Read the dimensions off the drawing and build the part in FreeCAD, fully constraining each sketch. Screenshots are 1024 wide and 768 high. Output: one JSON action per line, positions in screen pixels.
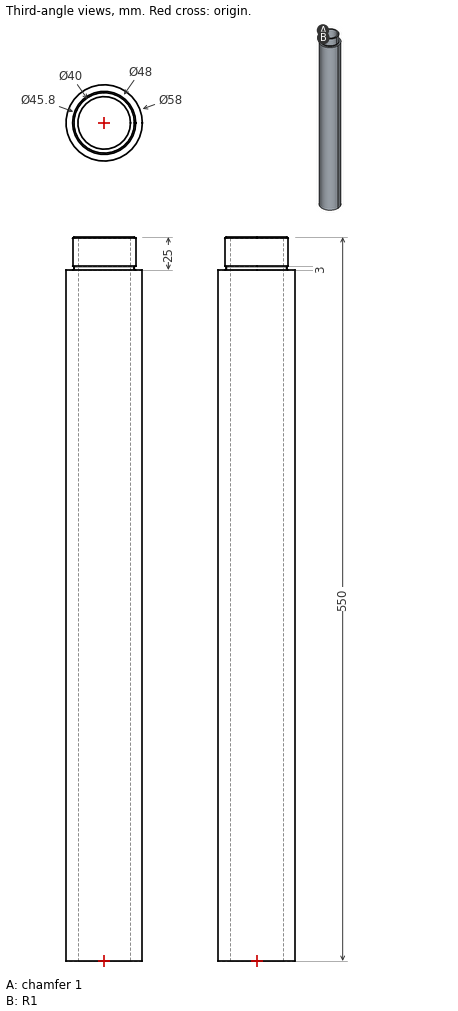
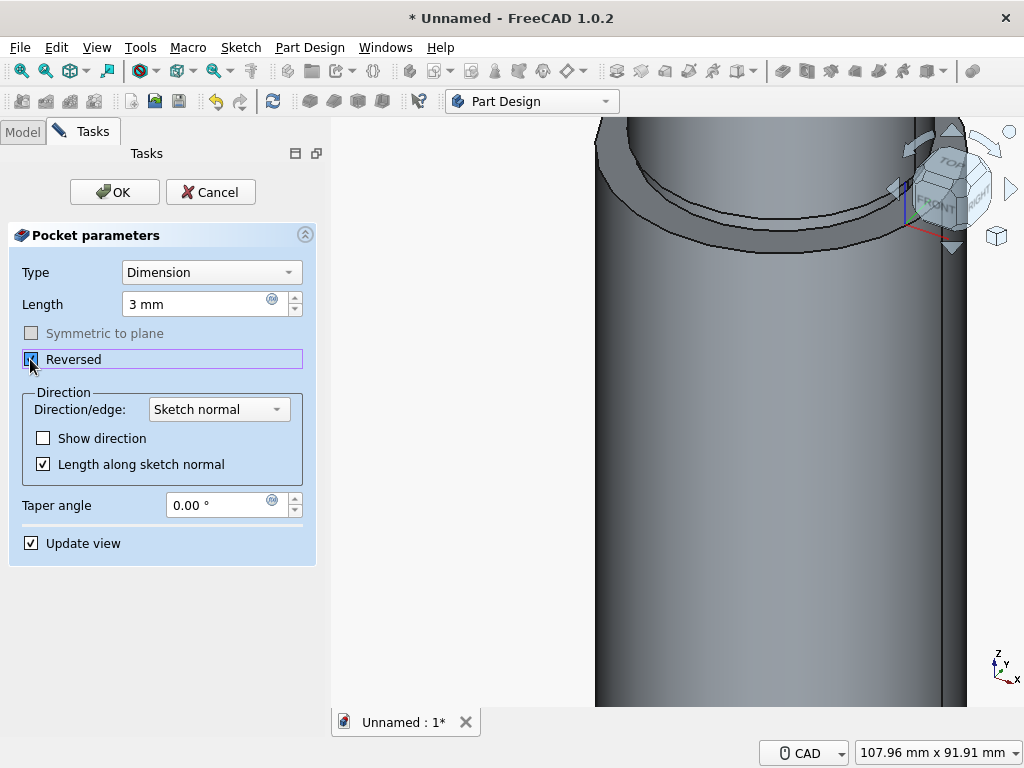
{"action": "left_click", "coordinate": [115, 192]}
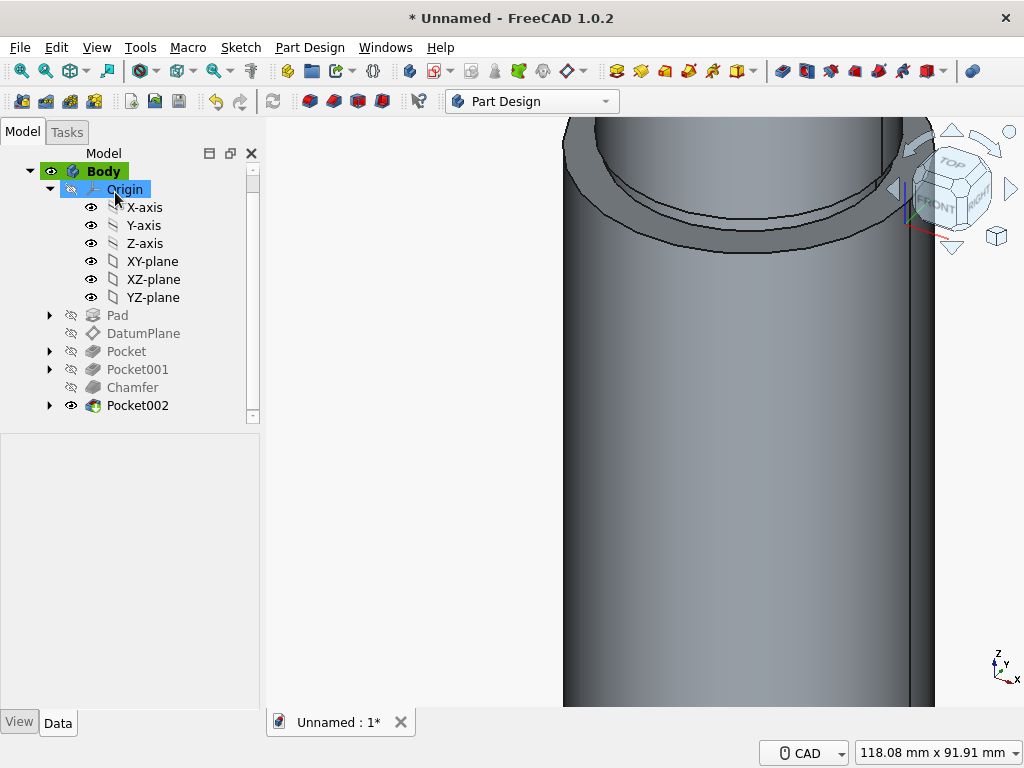
{"action": "left_click", "coordinate": [22, 72]}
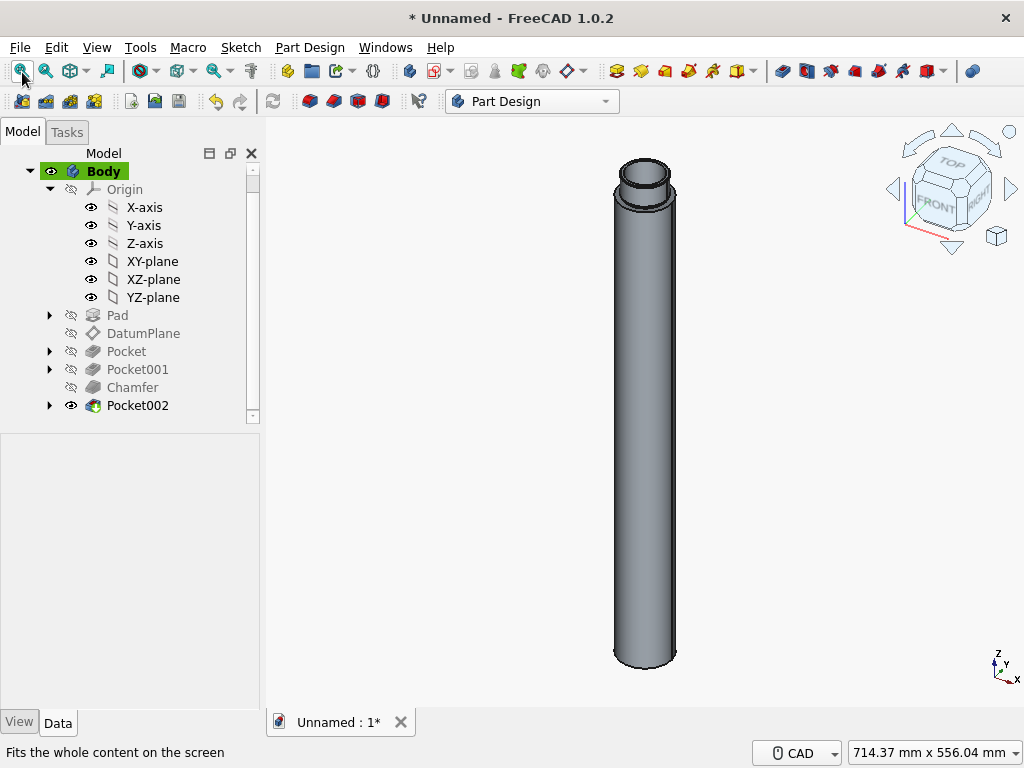
{"action": "key", "text": "0"}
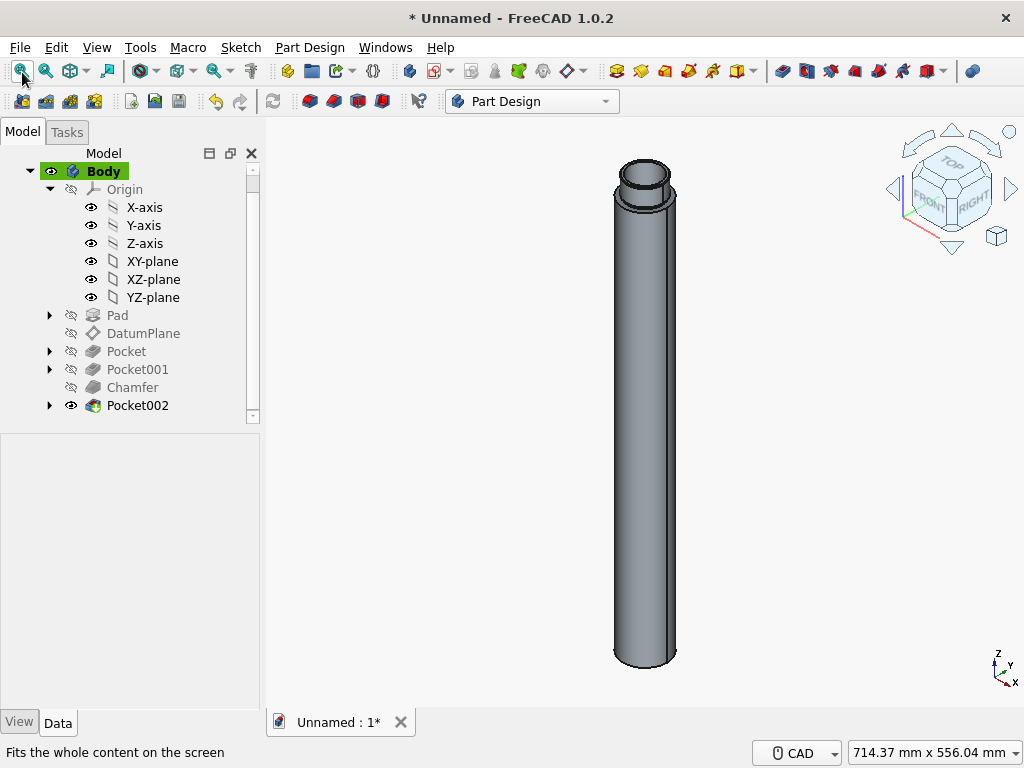
{"action": "key", "text": "2"}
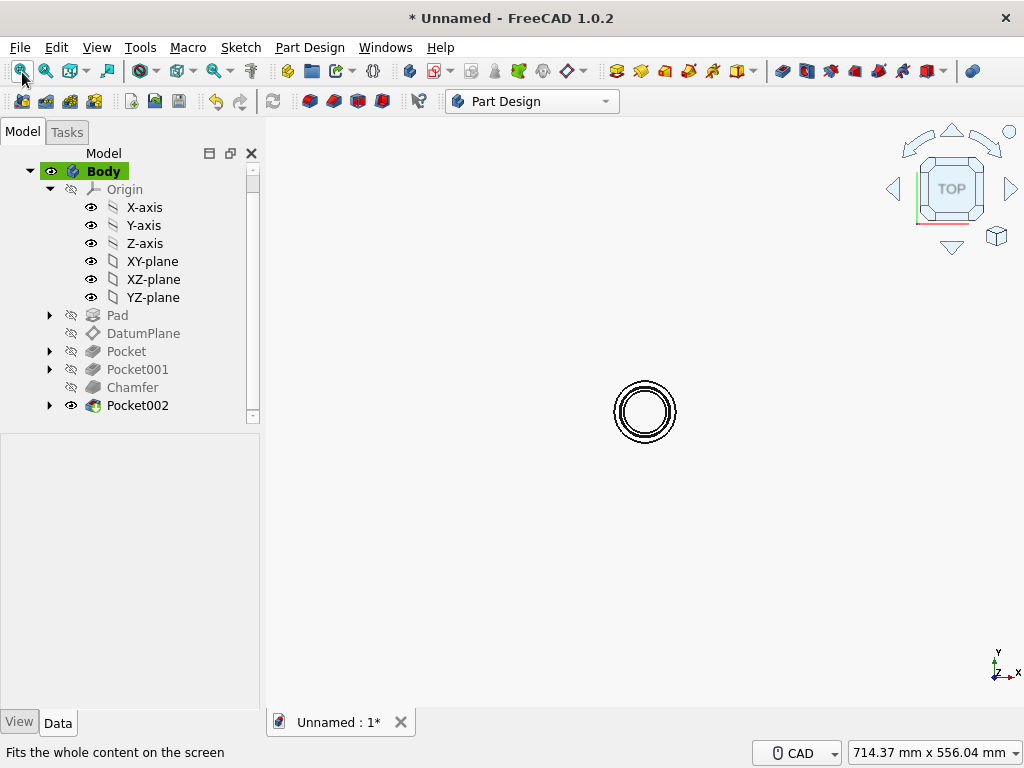
{"action": "left_click", "coordinate": [22, 72]}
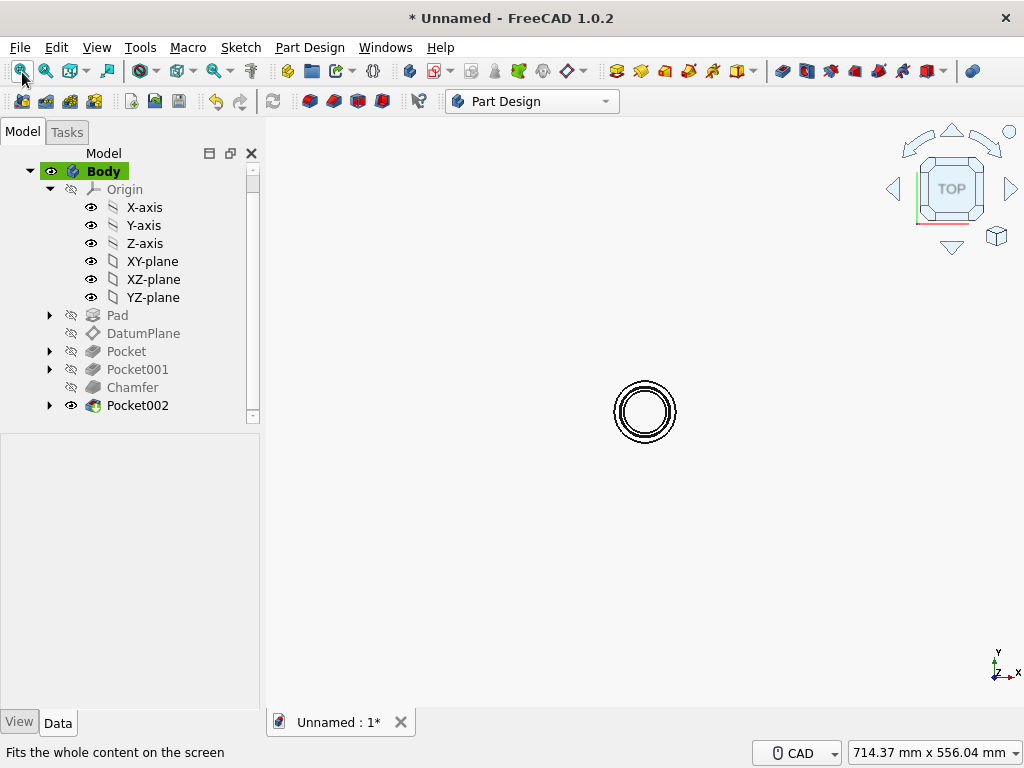
{"action": "key", "text": "1"}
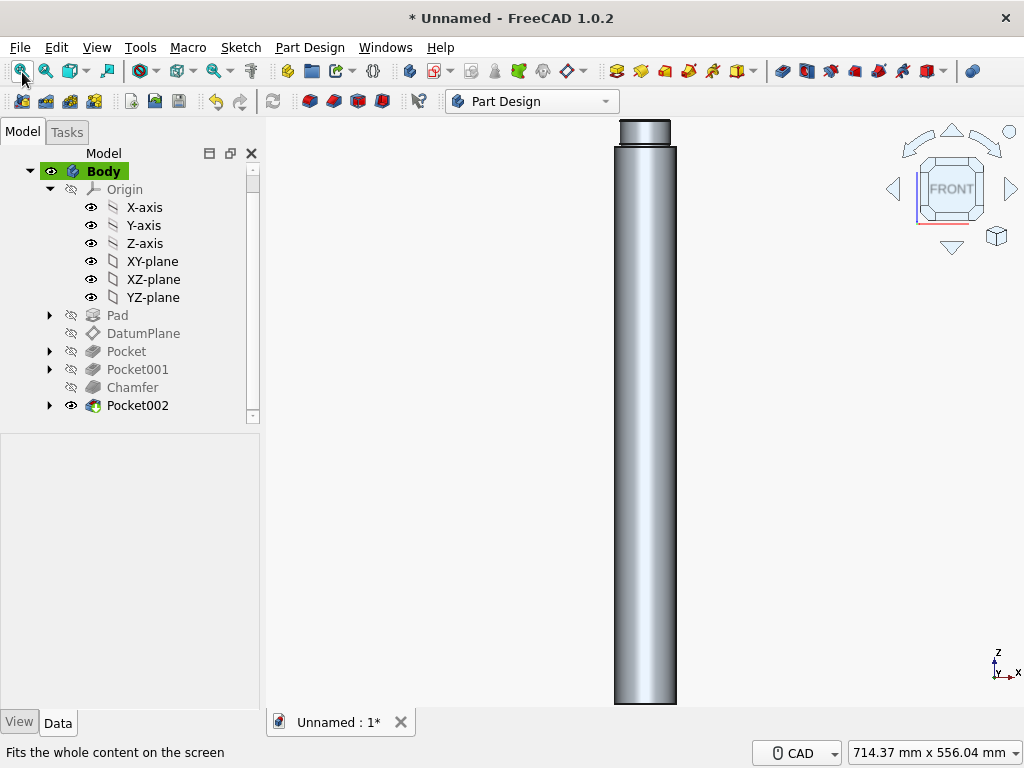
{"action": "key", "text": "3"}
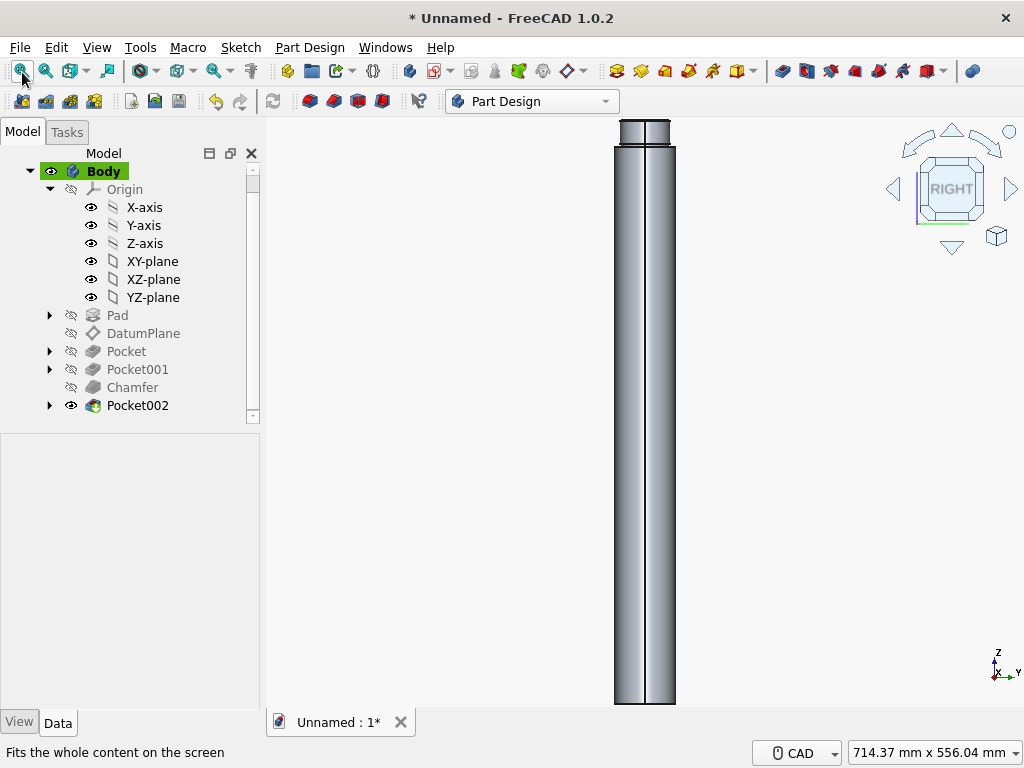
{"action": "key", "text": "5"}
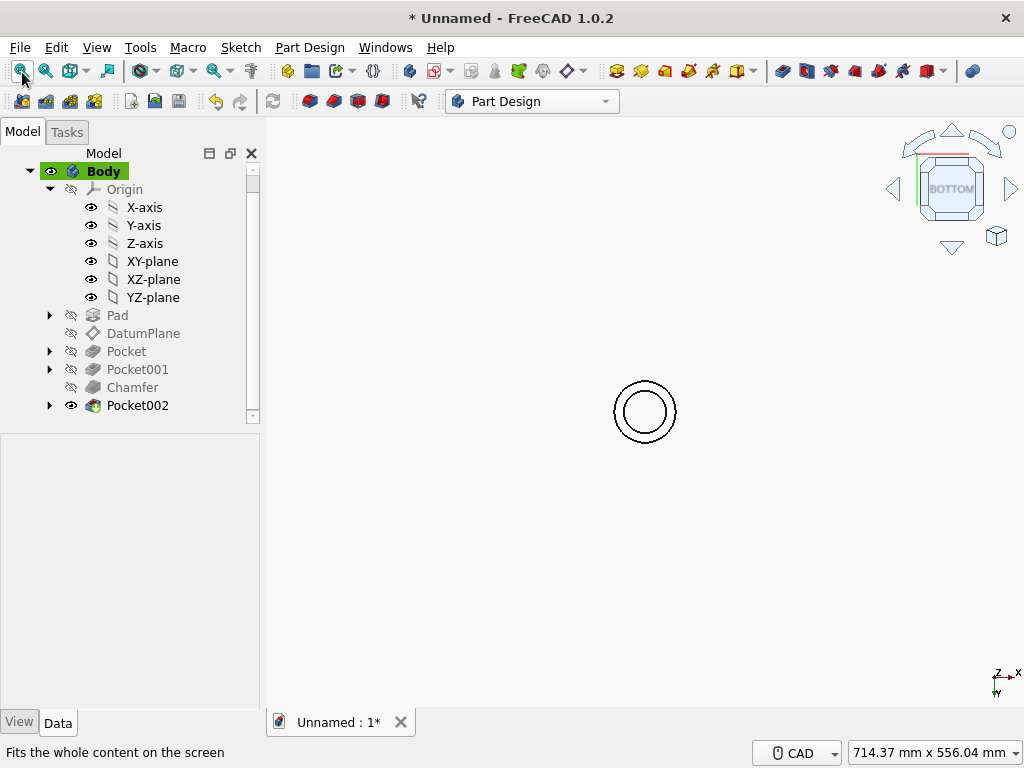
{"action": "left_click", "coordinate": [22, 72]}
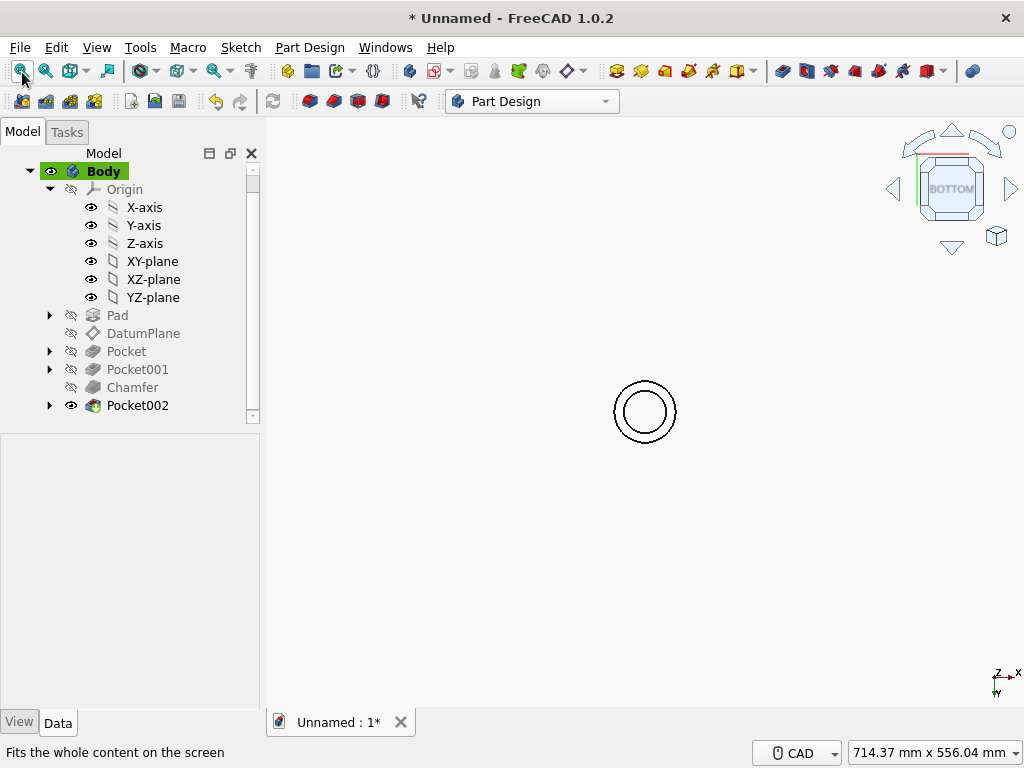
{"action": "key", "text": "4"}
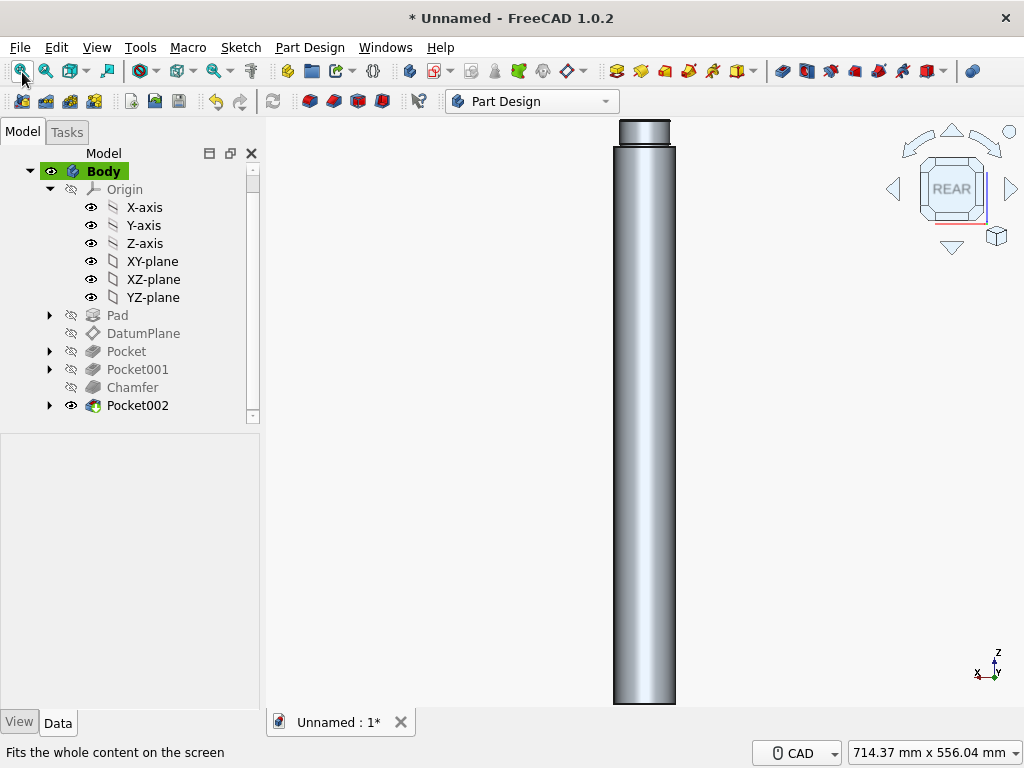
{"action": "key", "text": "6"}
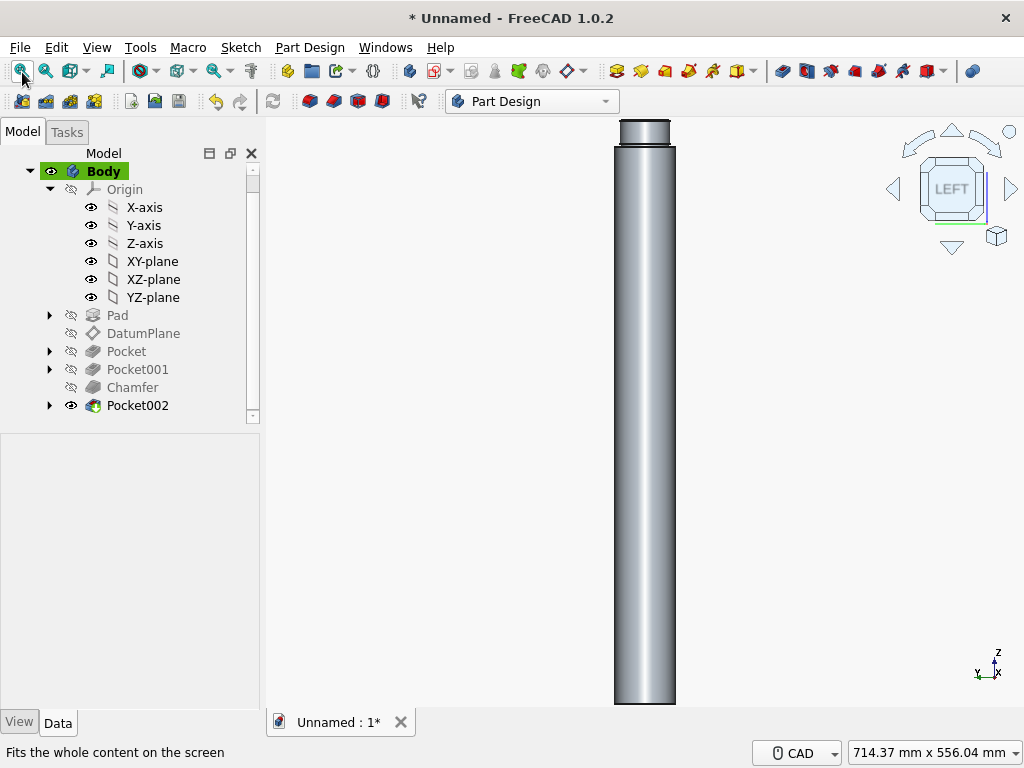
{"action": "key", "text": "v 3"}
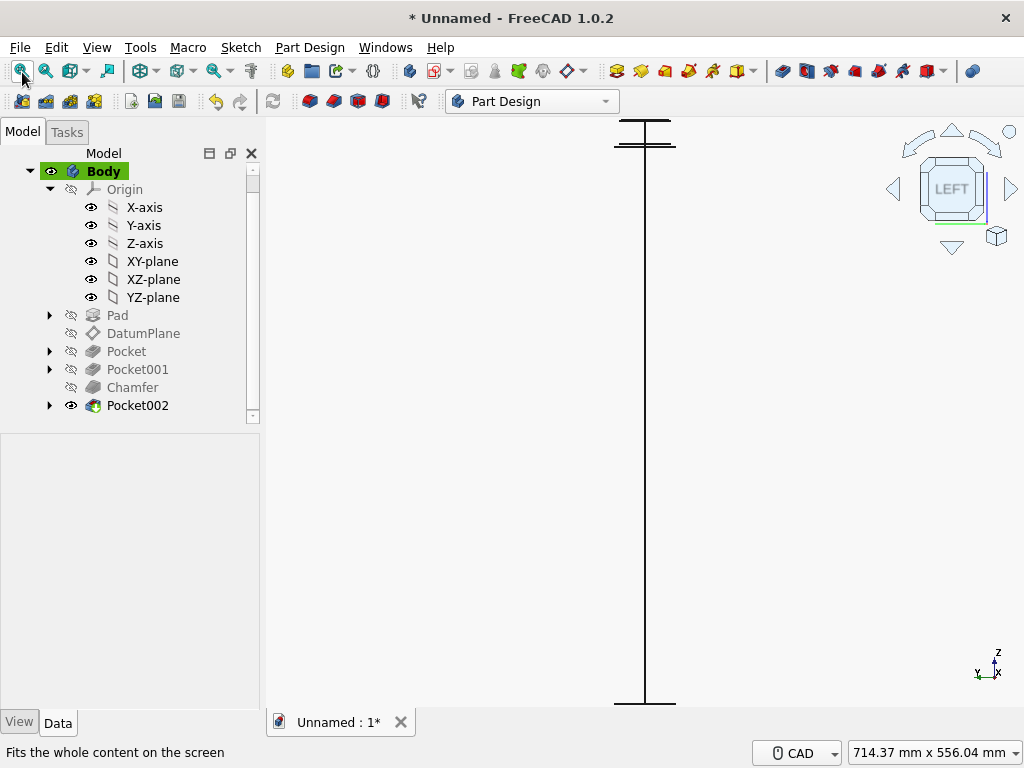
{"action": "key", "text": "0"}